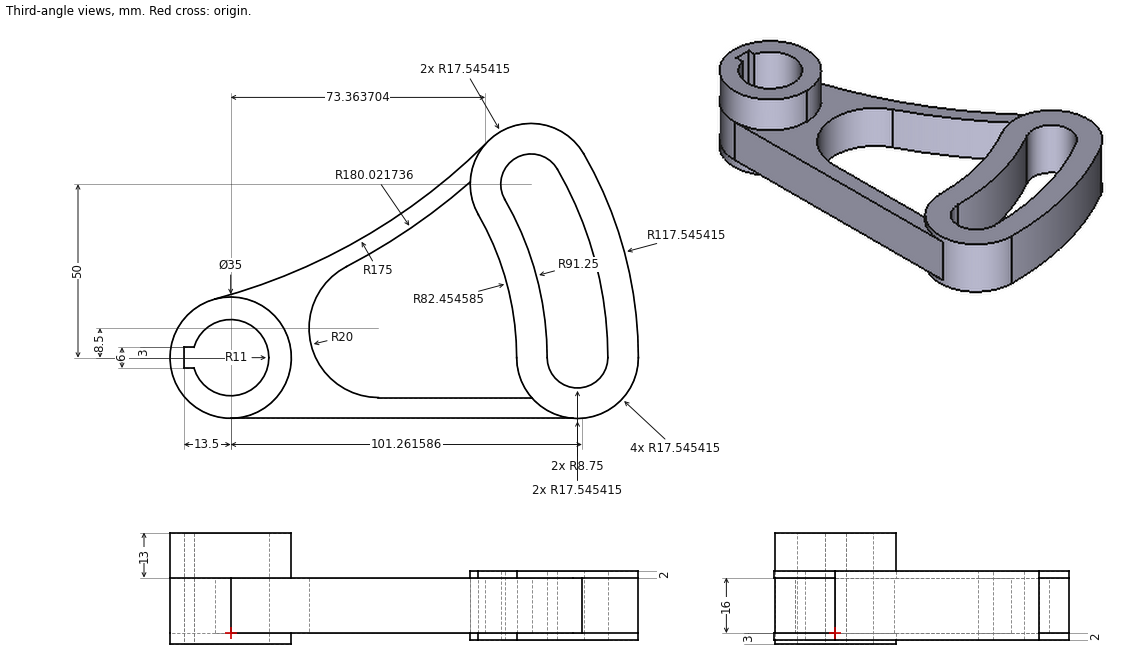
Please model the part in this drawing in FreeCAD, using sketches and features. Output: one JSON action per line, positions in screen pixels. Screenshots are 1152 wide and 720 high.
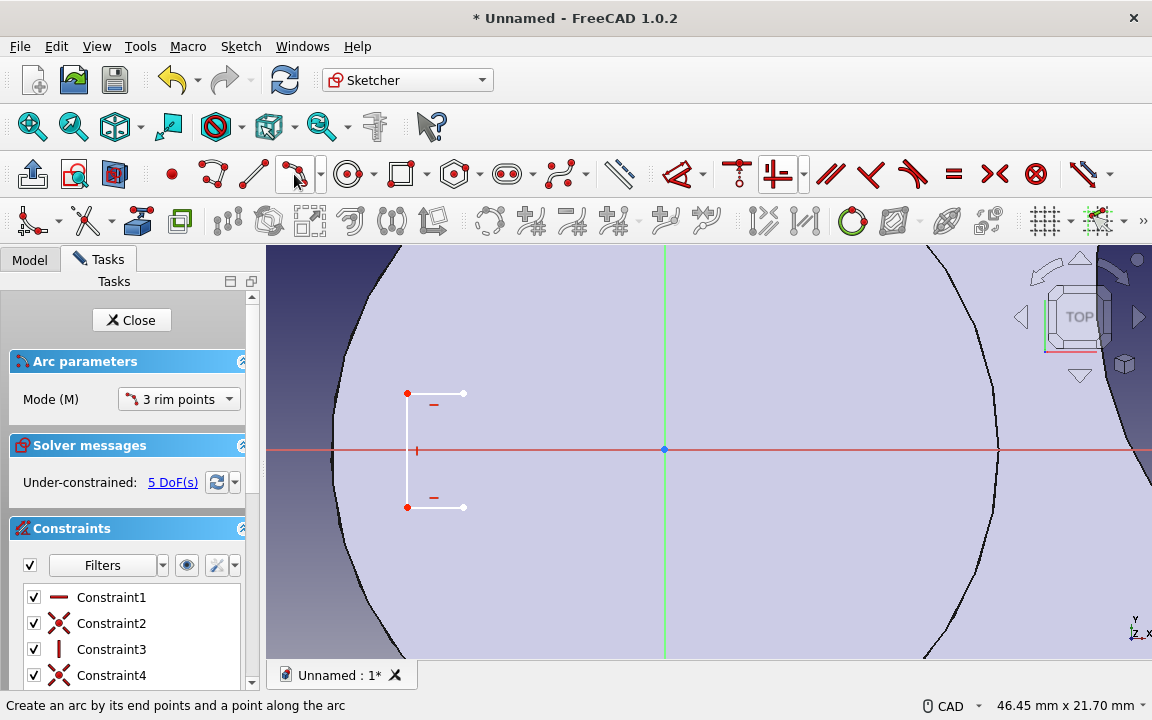
{"action": "left_click", "coordinate": [463, 508]}
{"action": "left_click", "coordinate": [463, 394]}
{"action": "left_click", "coordinate": [841, 564]}
{"action": "key", "text": "Escape"}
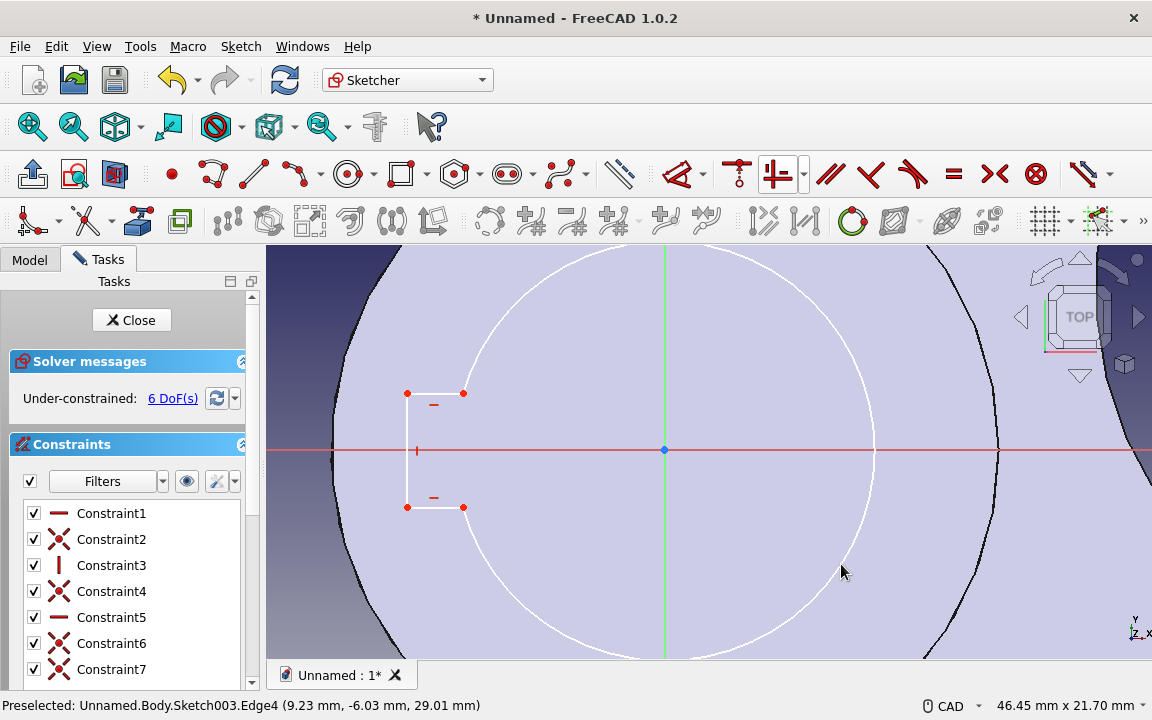
{"action": "left_click_drag", "start_coordinate": [655, 440], "coordinate": [675, 461]}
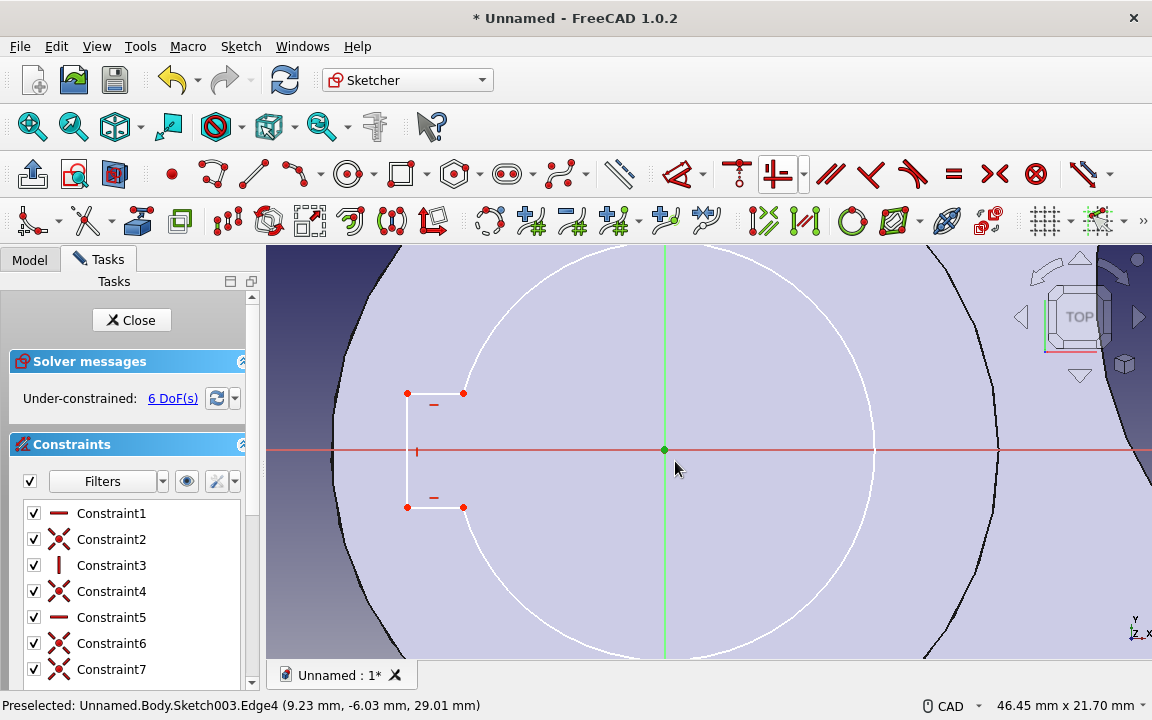
{"action": "left_click", "coordinate": [737, 174]}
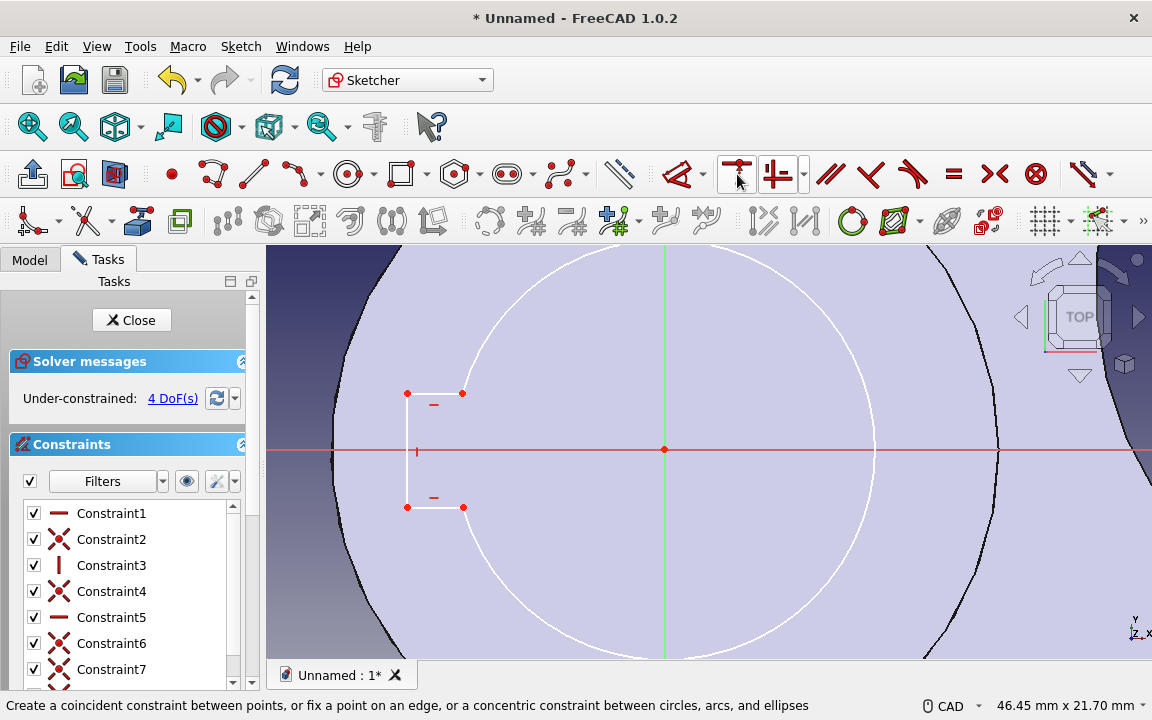
{"action": "left_click", "coordinate": [676, 174]}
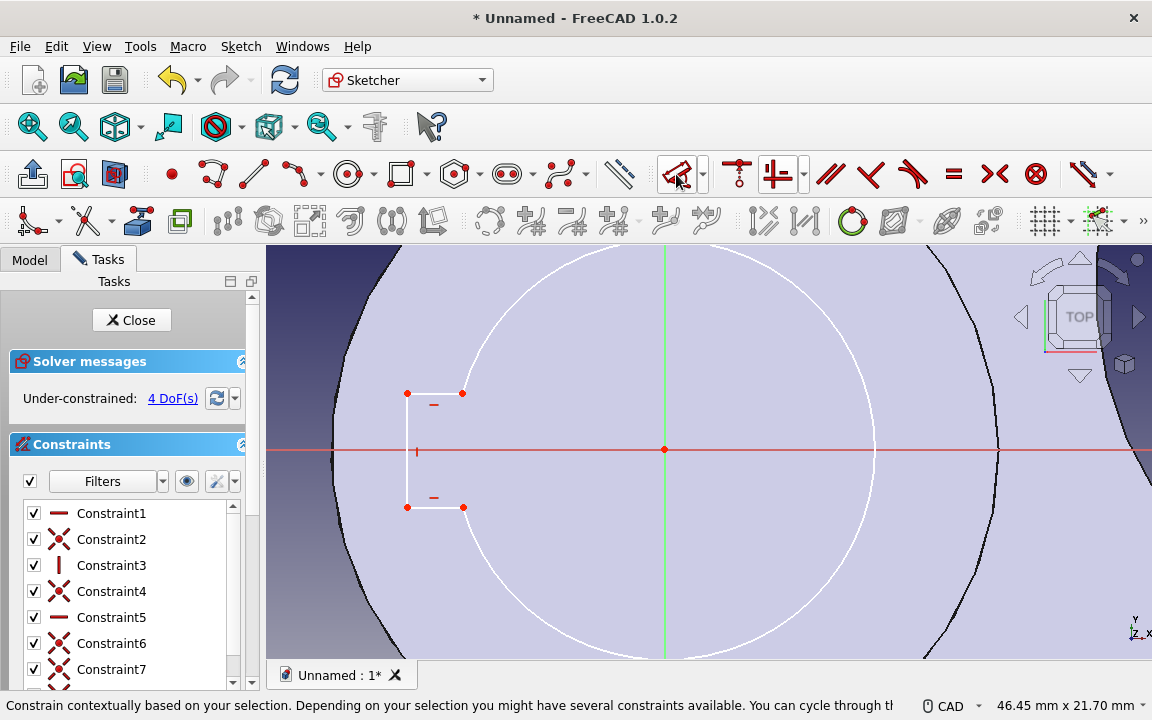
{"action": "left_click", "coordinate": [875, 449]}
{"action": "left_click", "coordinate": [878, 565]}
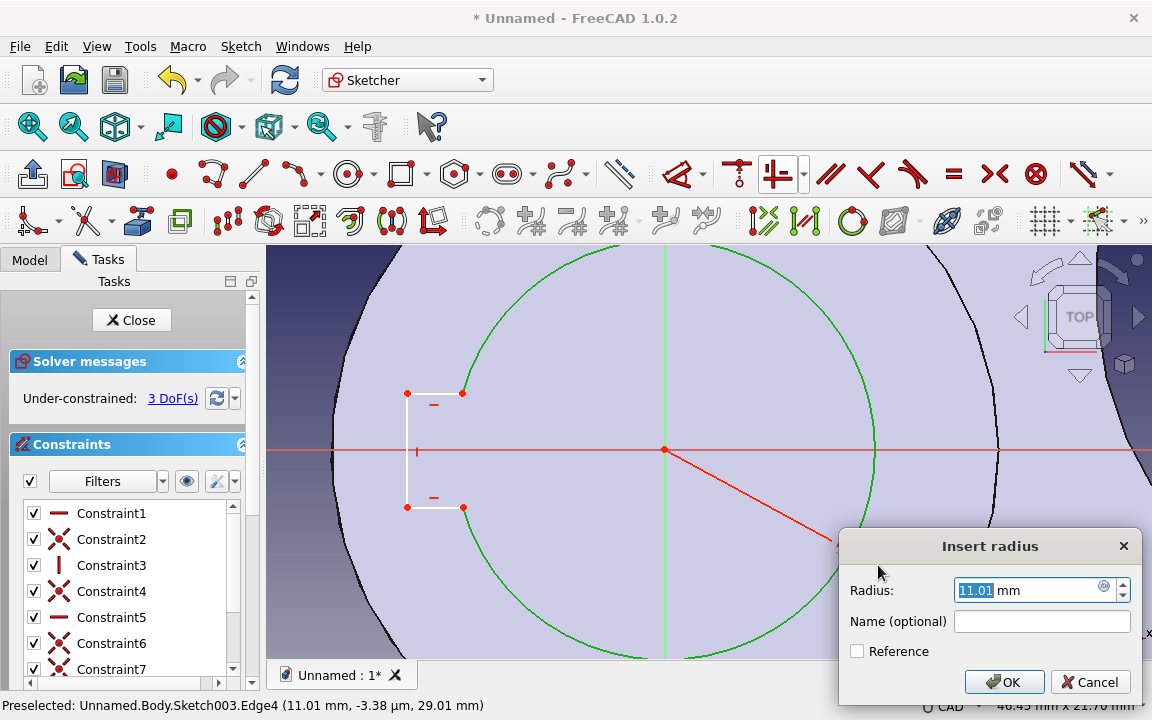
{"action": "type", "text": "11"}
{"action": "key", "text": "Return"}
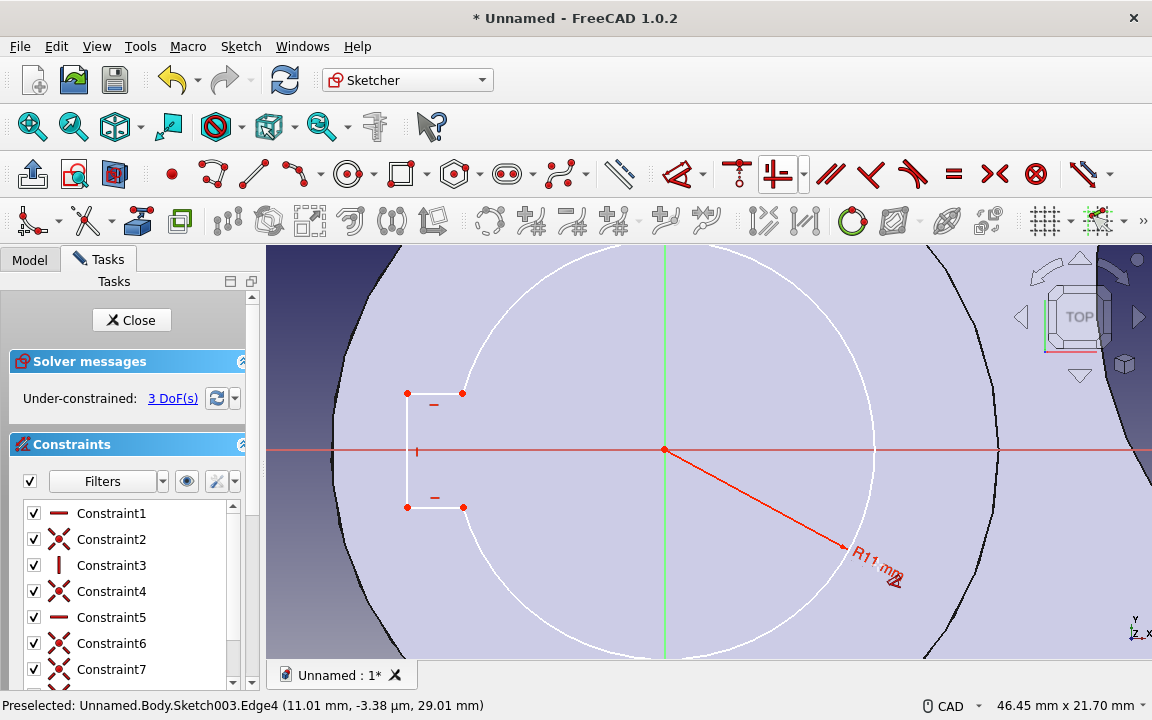
{"action": "left_click", "coordinate": [407, 428]}
{"action": "left_click", "coordinate": [373, 425]}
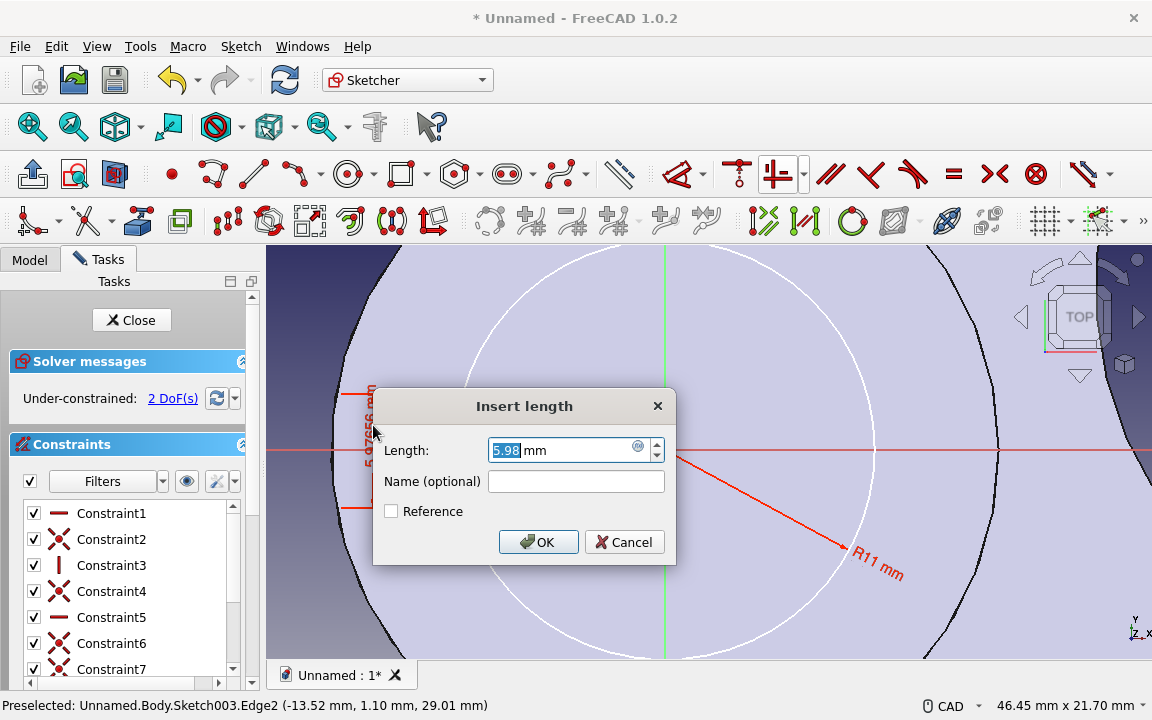
{"action": "type", "text": "6"}
{"action": "key", "text": "Return"}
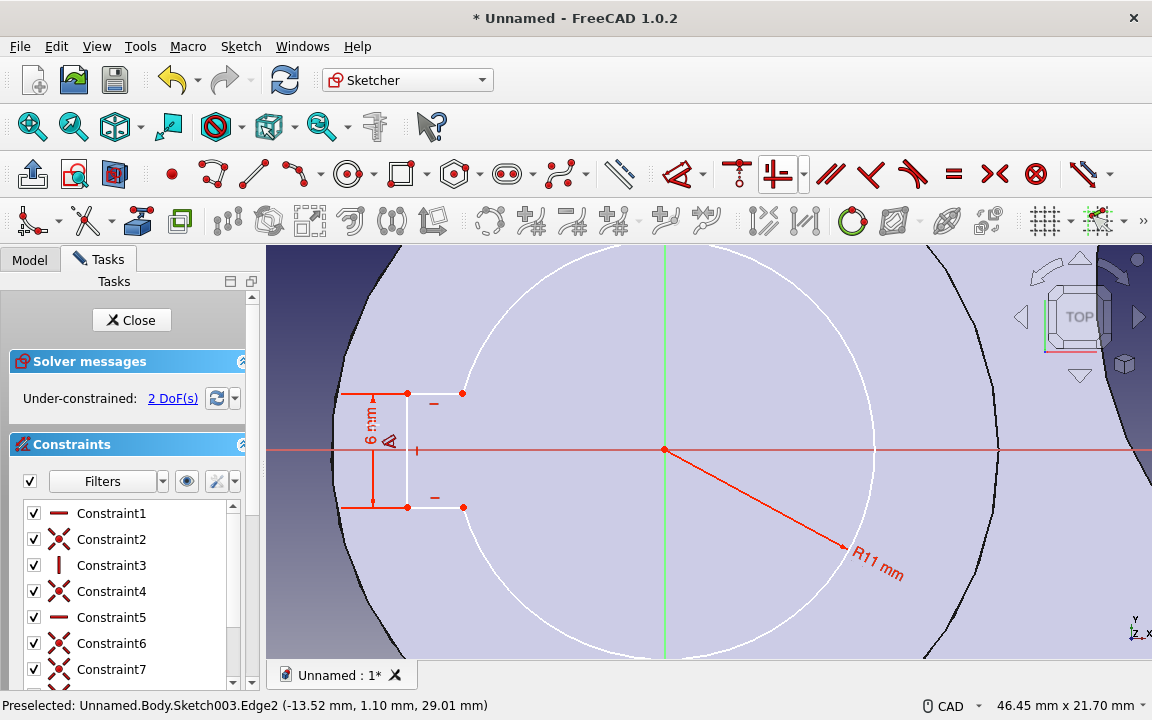
{"action": "left_click", "coordinate": [463, 394]}
{"action": "left_click", "coordinate": [699, 422]}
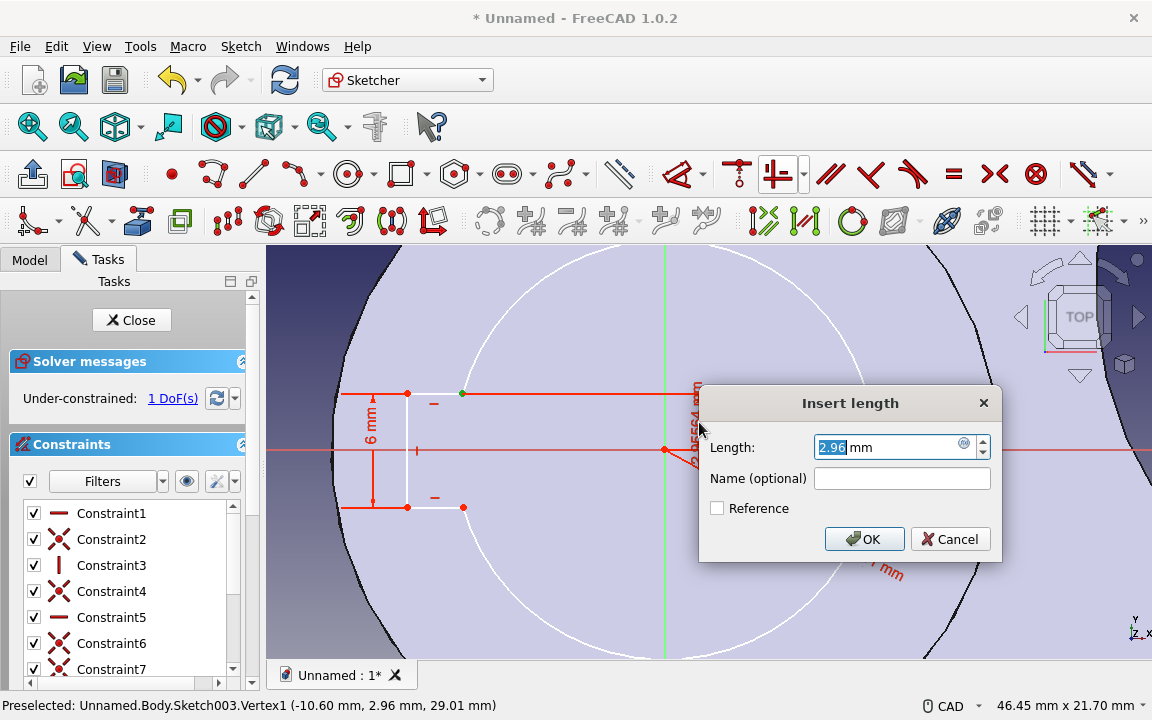
{"action": "type", "text": "3"}
{"action": "key", "text": "Return"}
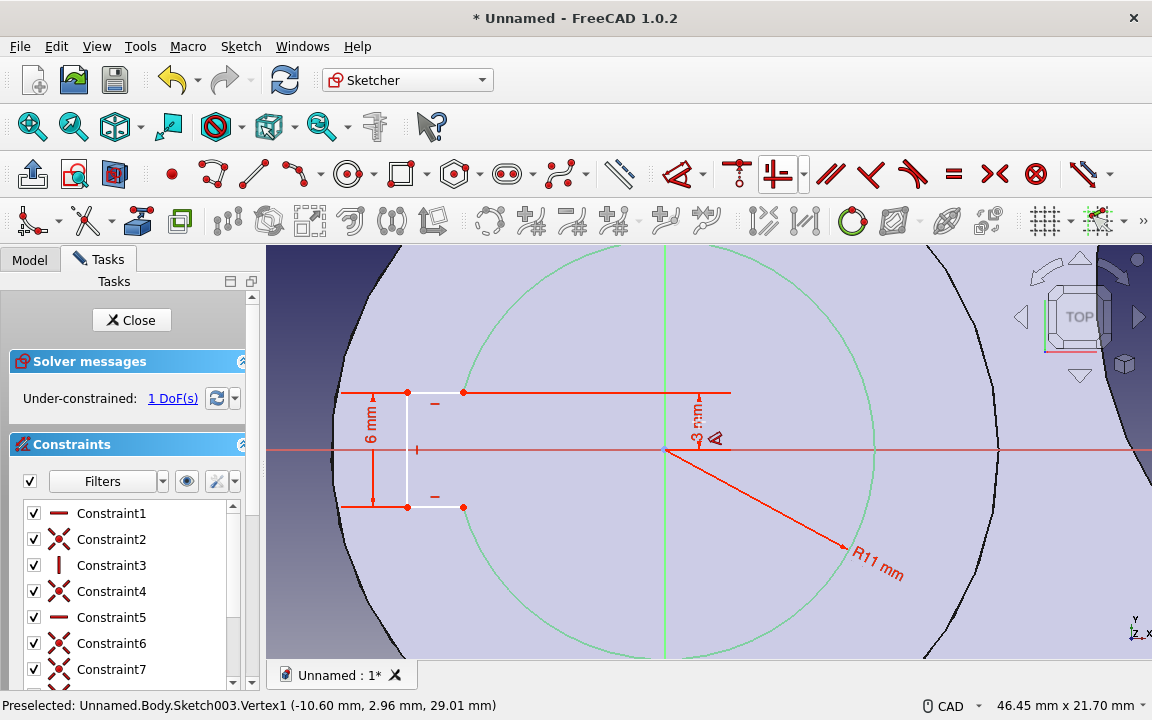
{"action": "left_click", "coordinate": [407, 393]}
{"action": "left_click", "coordinate": [536, 359]}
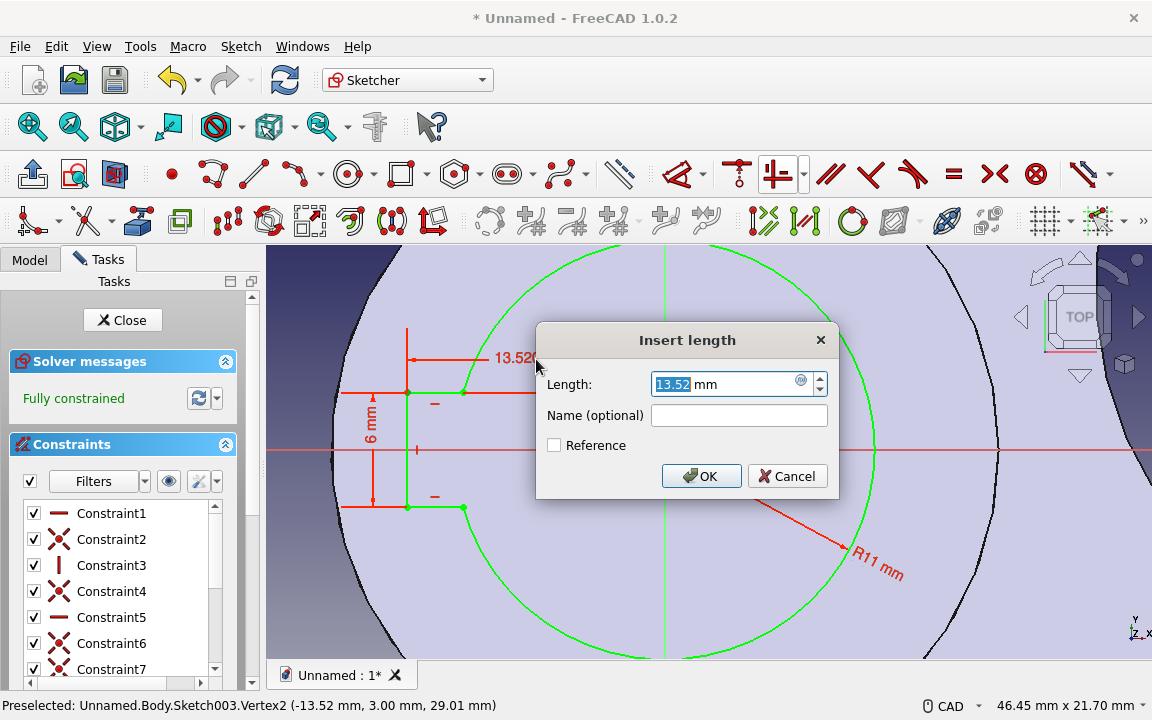
{"action": "type", "text": "13.5"}
{"action": "key", "text": "Return"}
{"action": "key", "text": "Escape"}